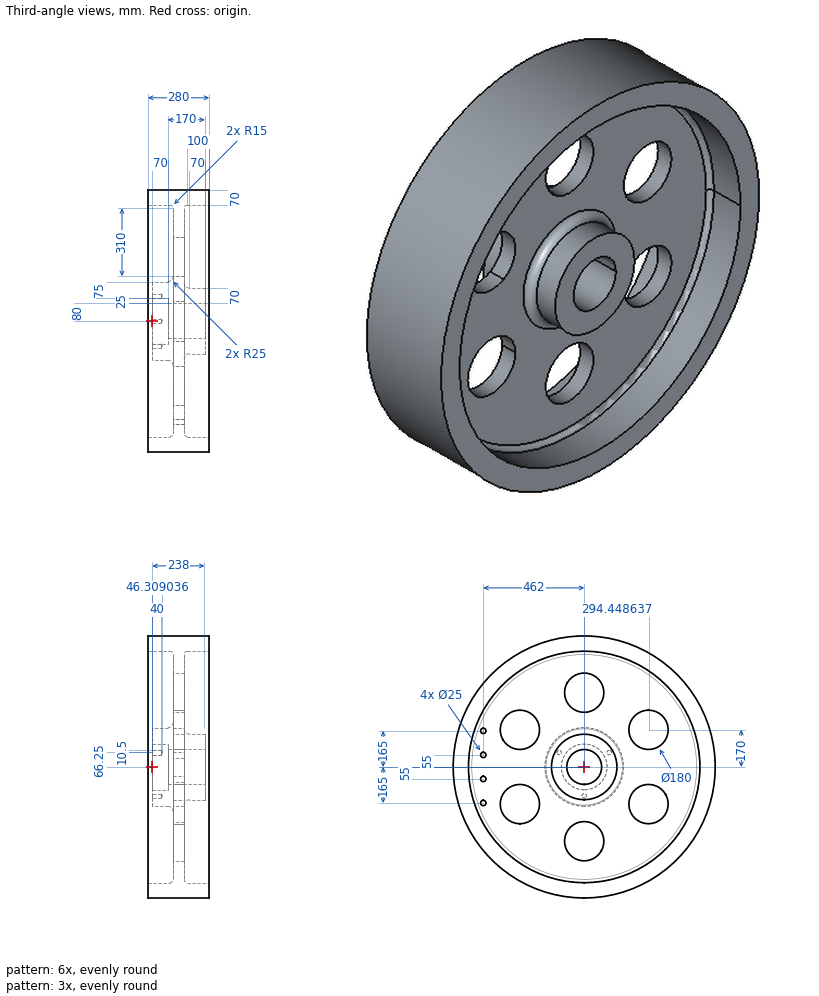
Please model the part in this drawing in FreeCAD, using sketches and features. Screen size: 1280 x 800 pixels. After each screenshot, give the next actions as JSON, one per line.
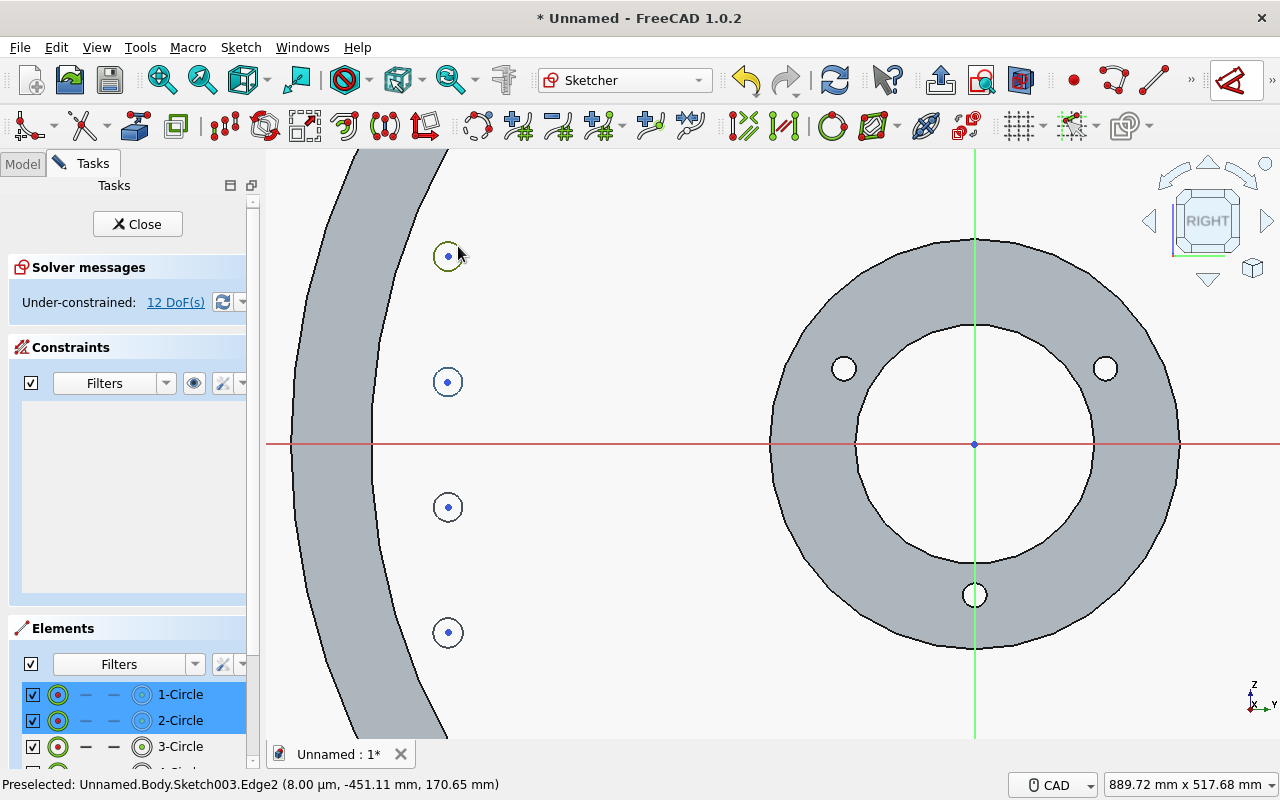
{"action": "left_click", "coordinate": [458, 497]}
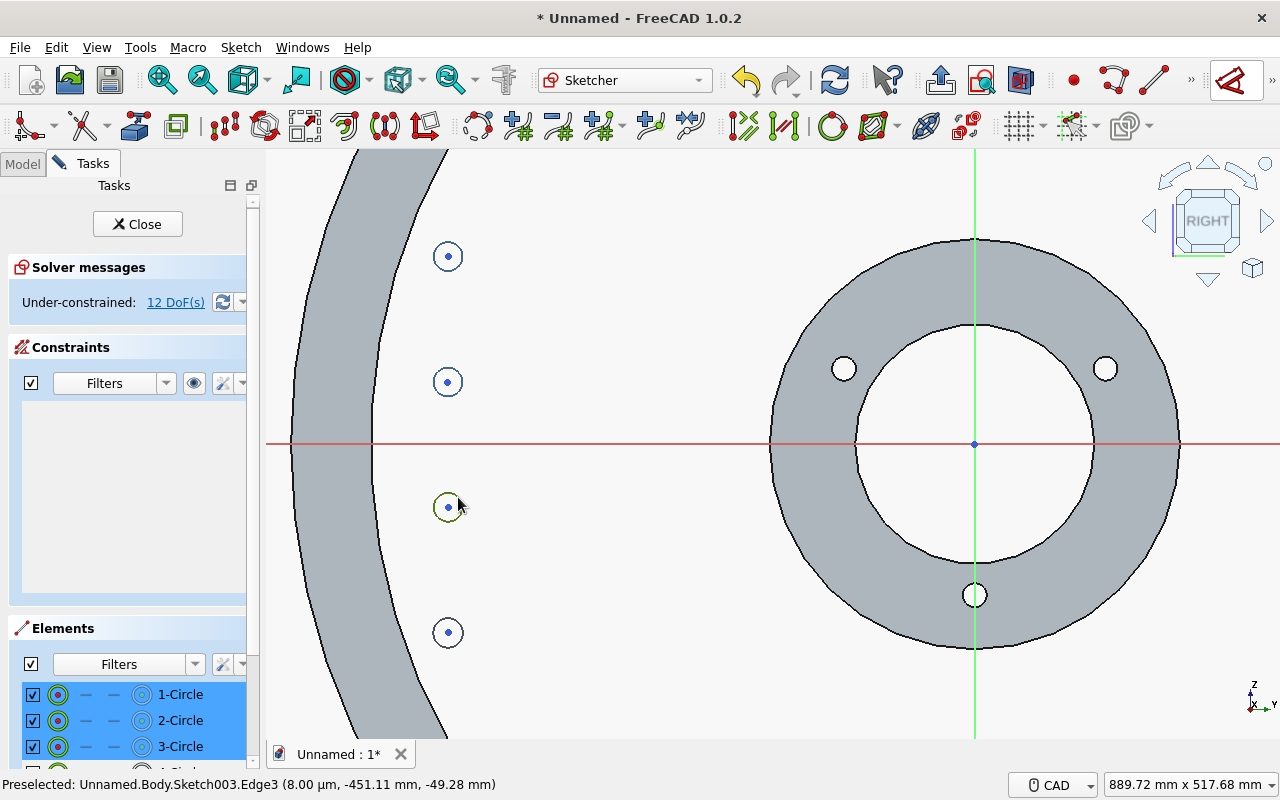
{"action": "left_click", "coordinate": [458, 622]}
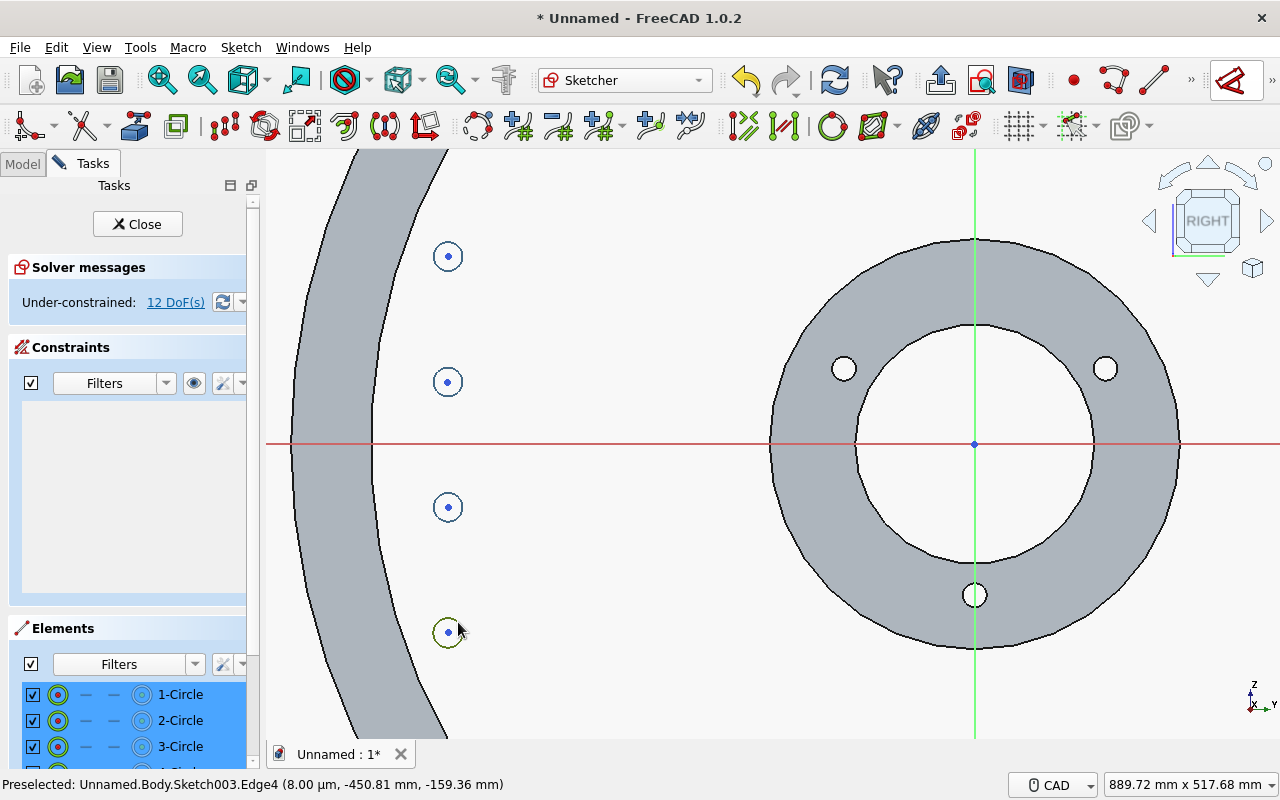
{"action": "key", "text": "e"}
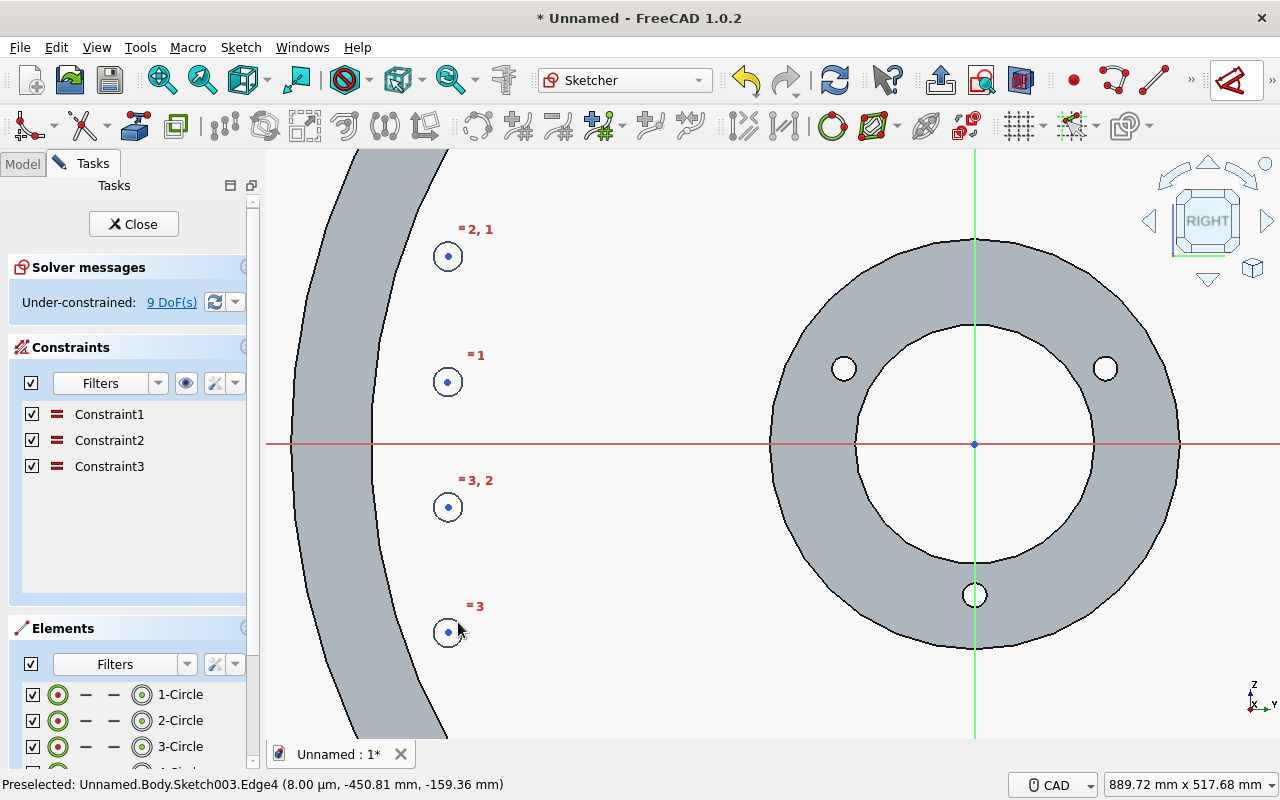
{"action": "left_click", "coordinate": [448, 382]}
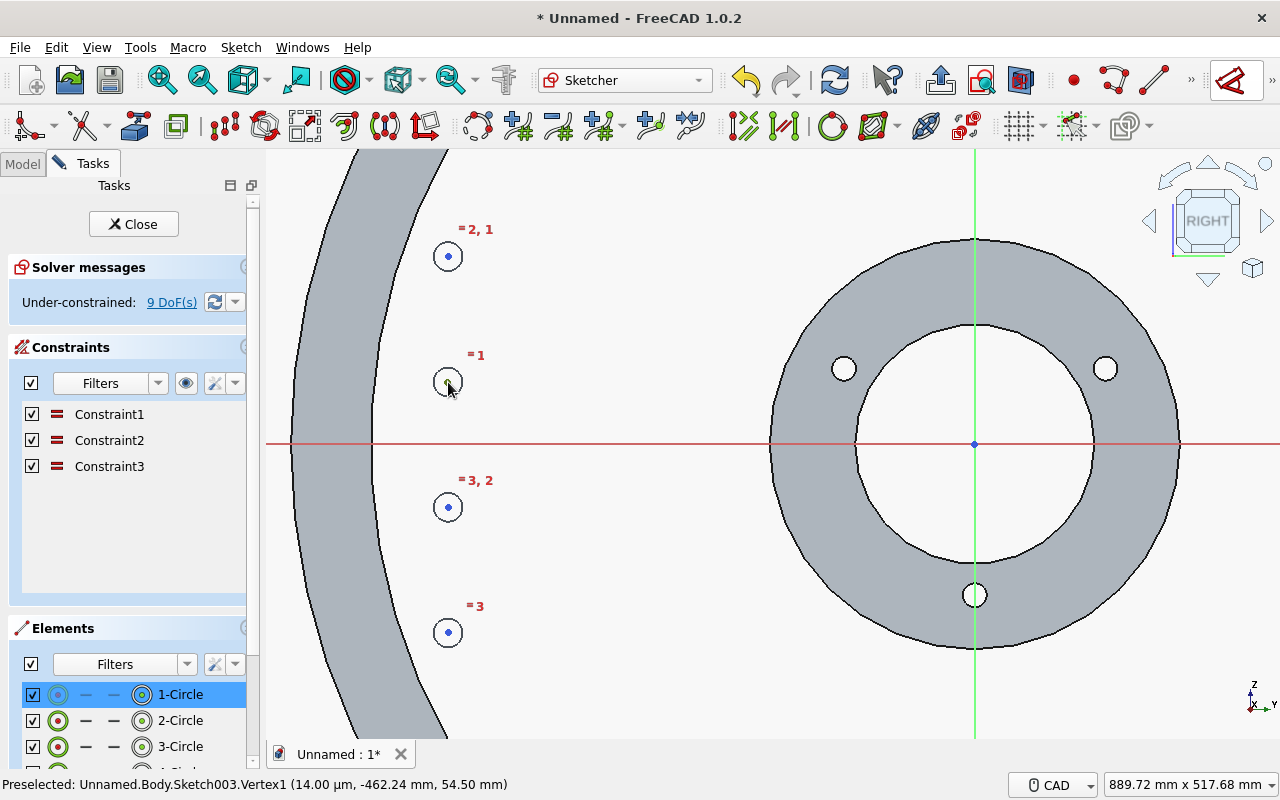
{"action": "left_click", "coordinate": [448, 257]}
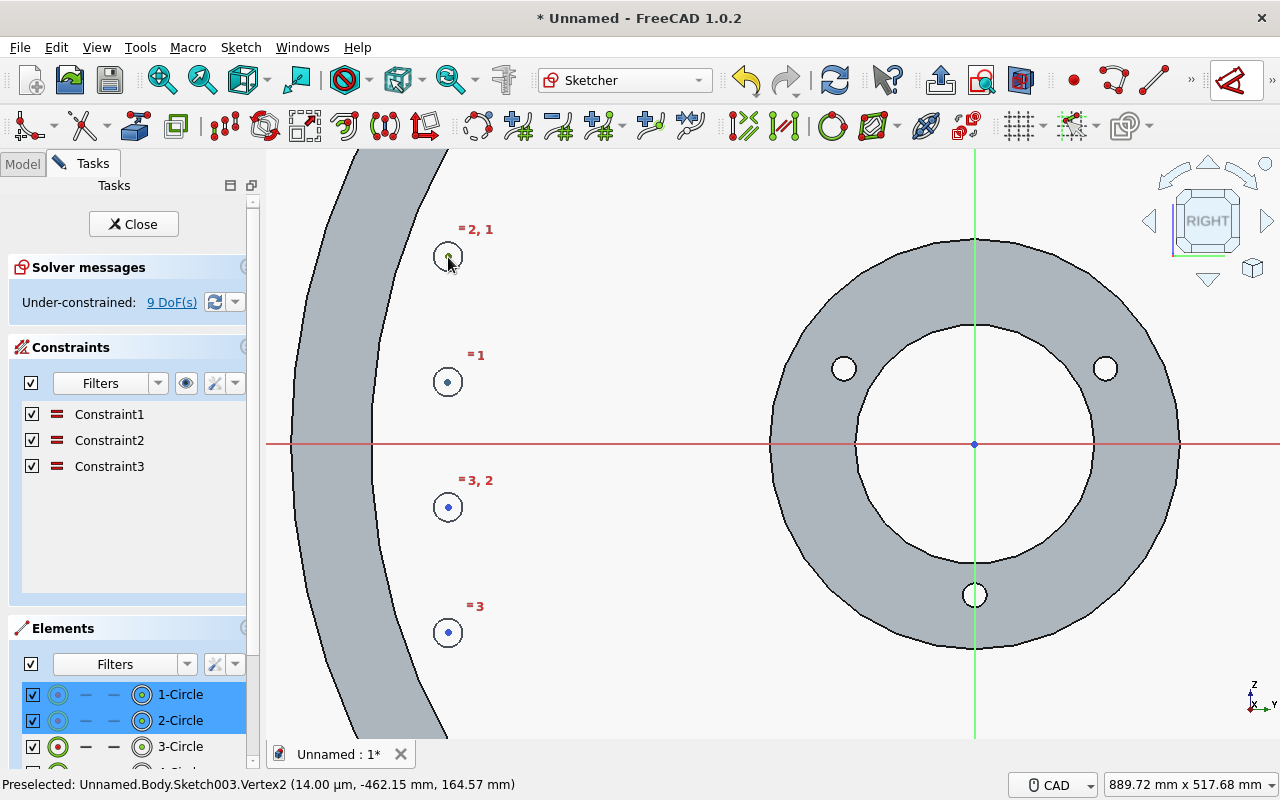
{"action": "key", "text": "v"}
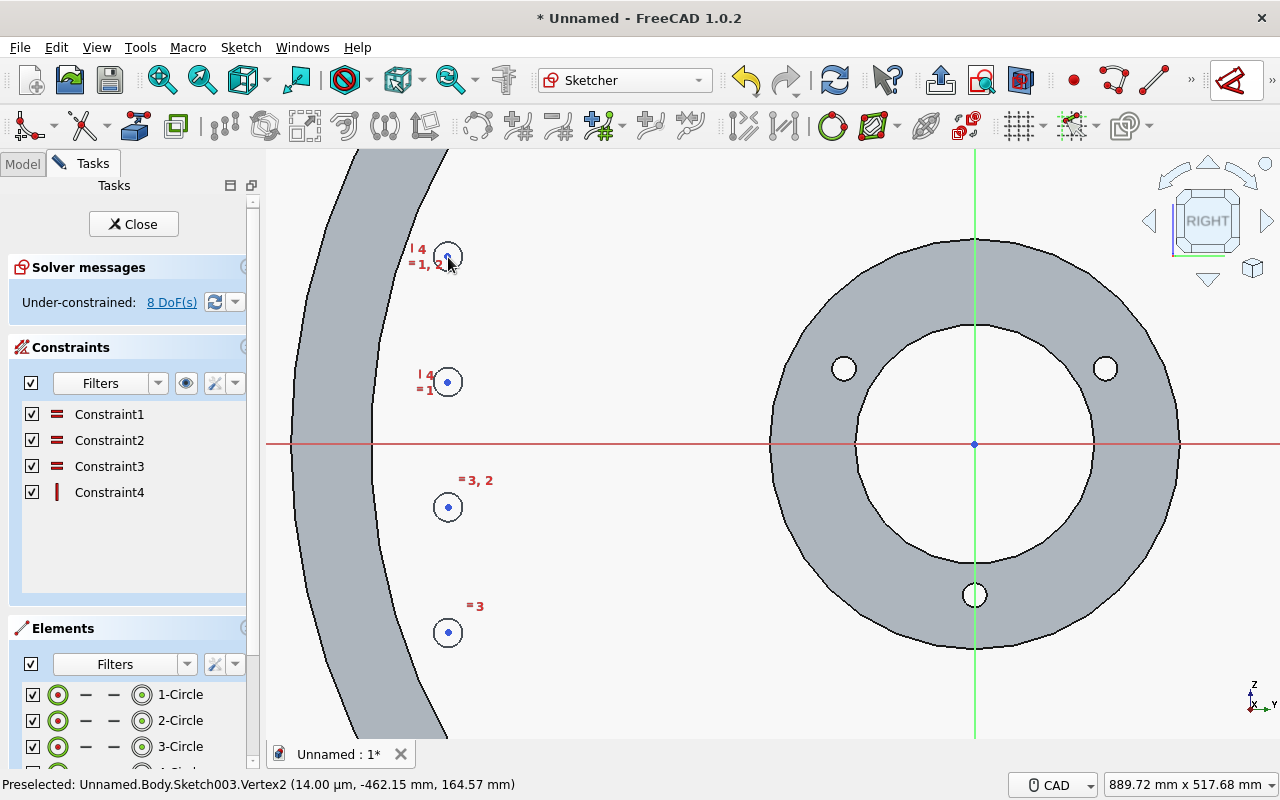
{"action": "left_click", "coordinate": [448, 382]}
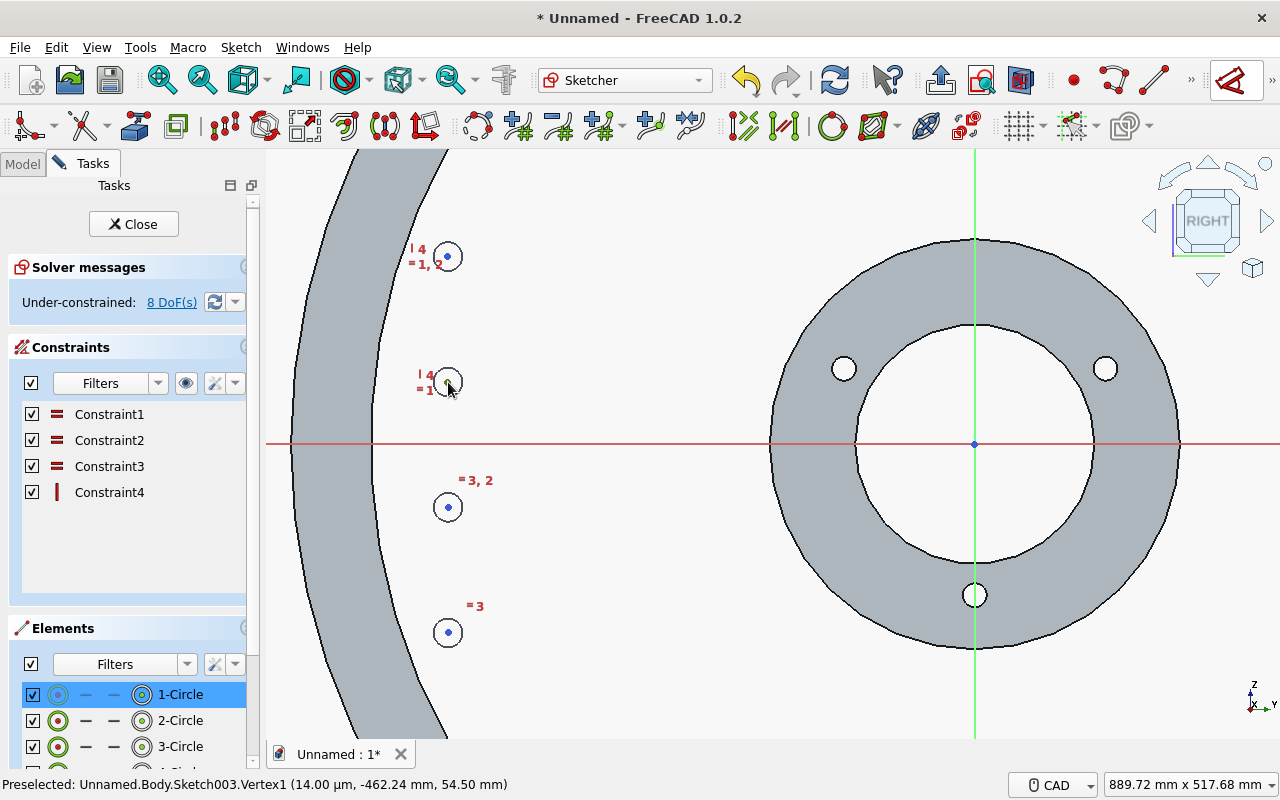
{"action": "left_click", "coordinate": [448, 507]}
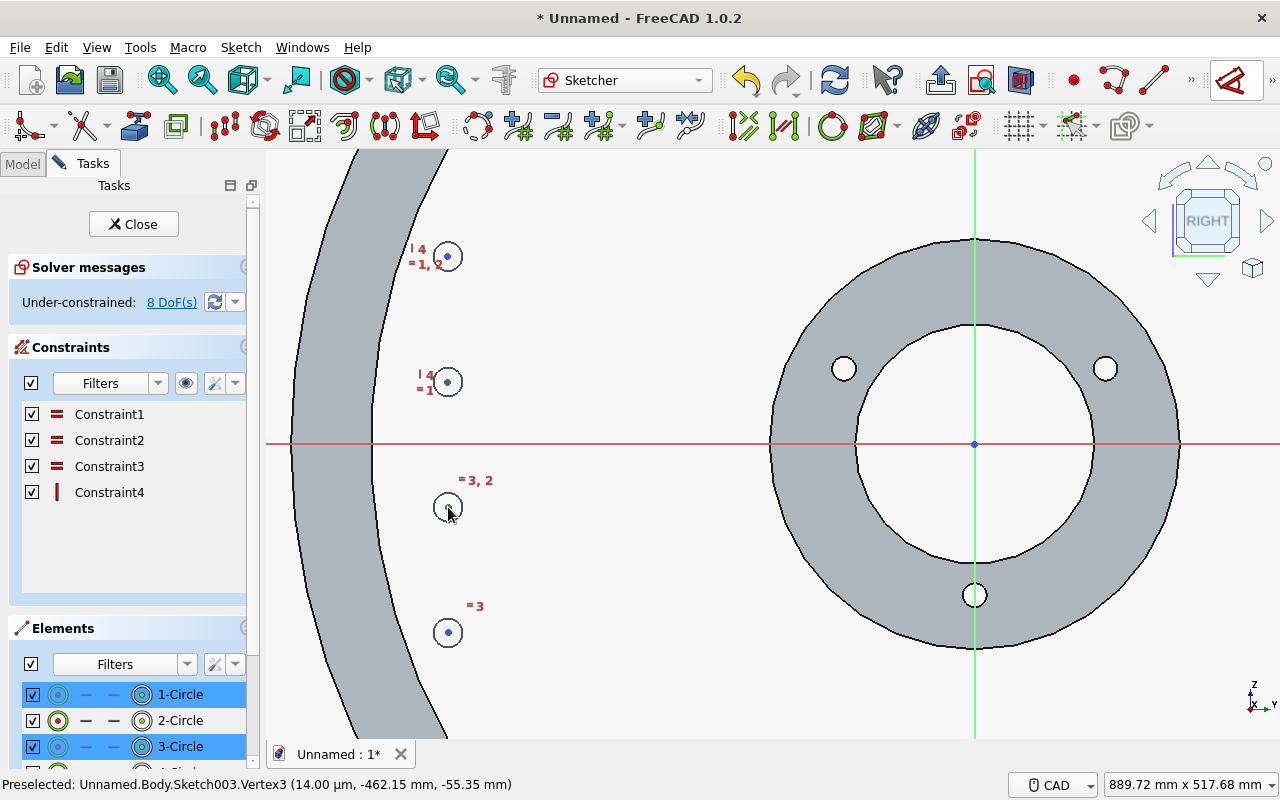
{"action": "key", "text": "v"}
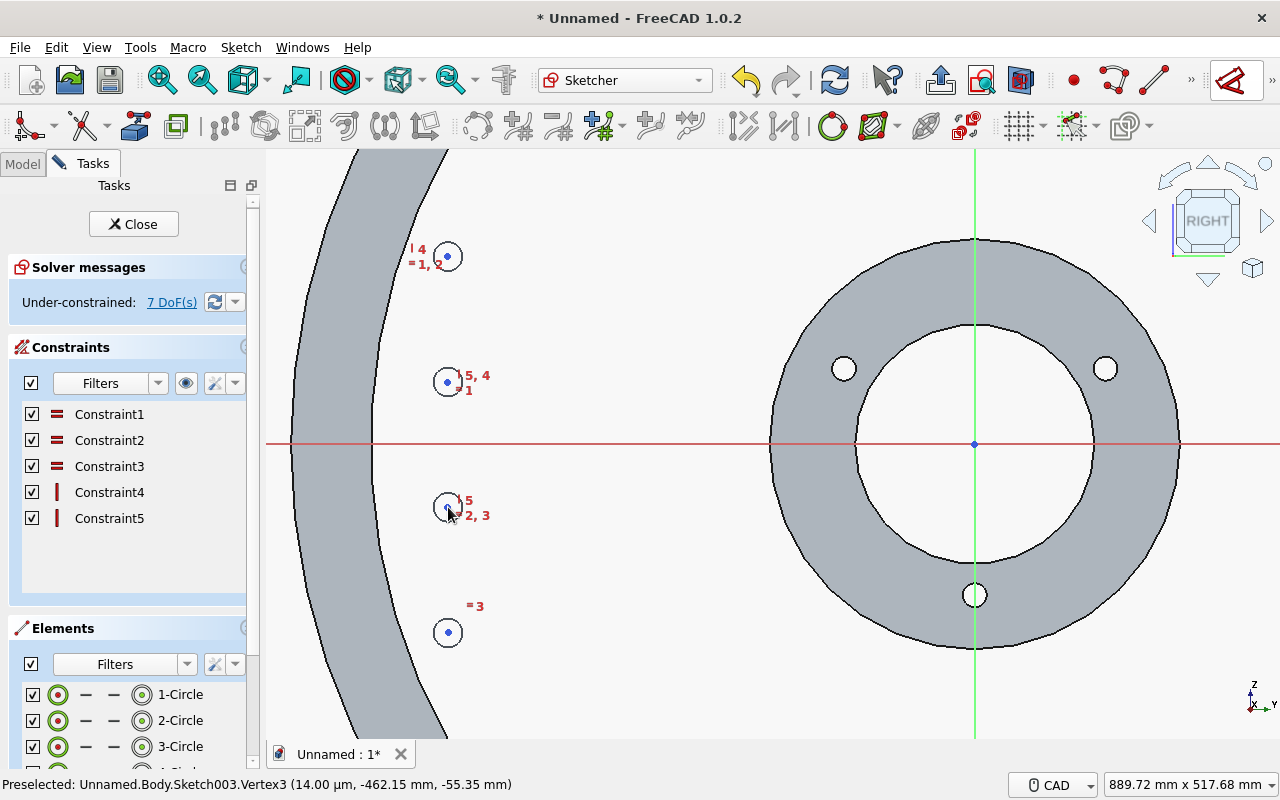
{"action": "left_click", "coordinate": [448, 507]}